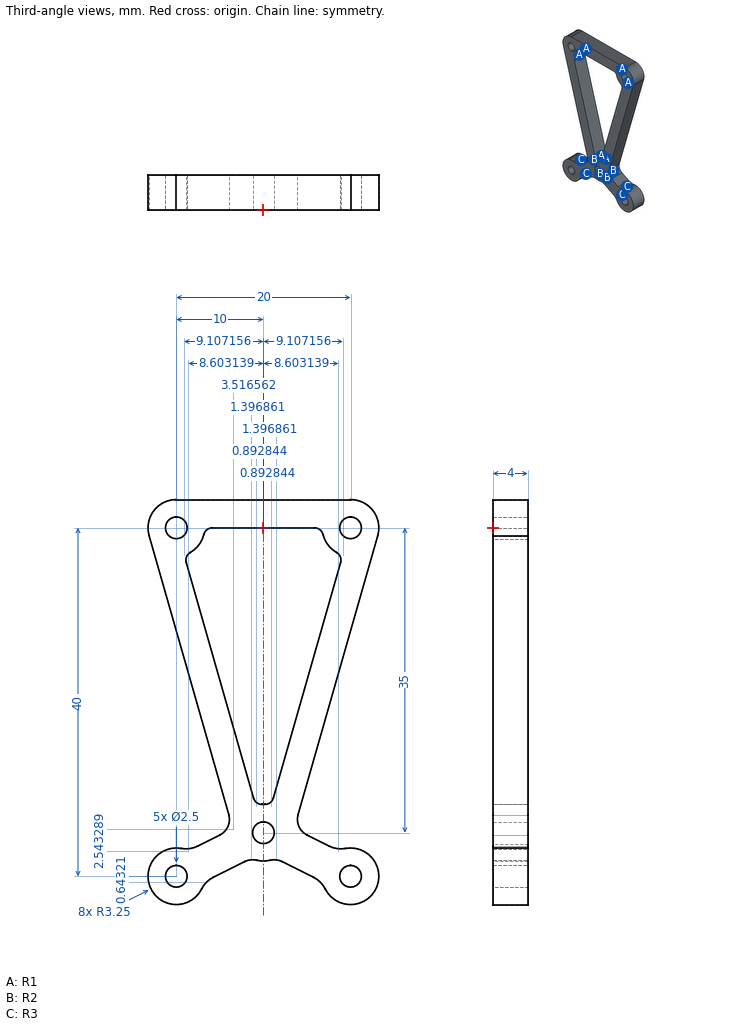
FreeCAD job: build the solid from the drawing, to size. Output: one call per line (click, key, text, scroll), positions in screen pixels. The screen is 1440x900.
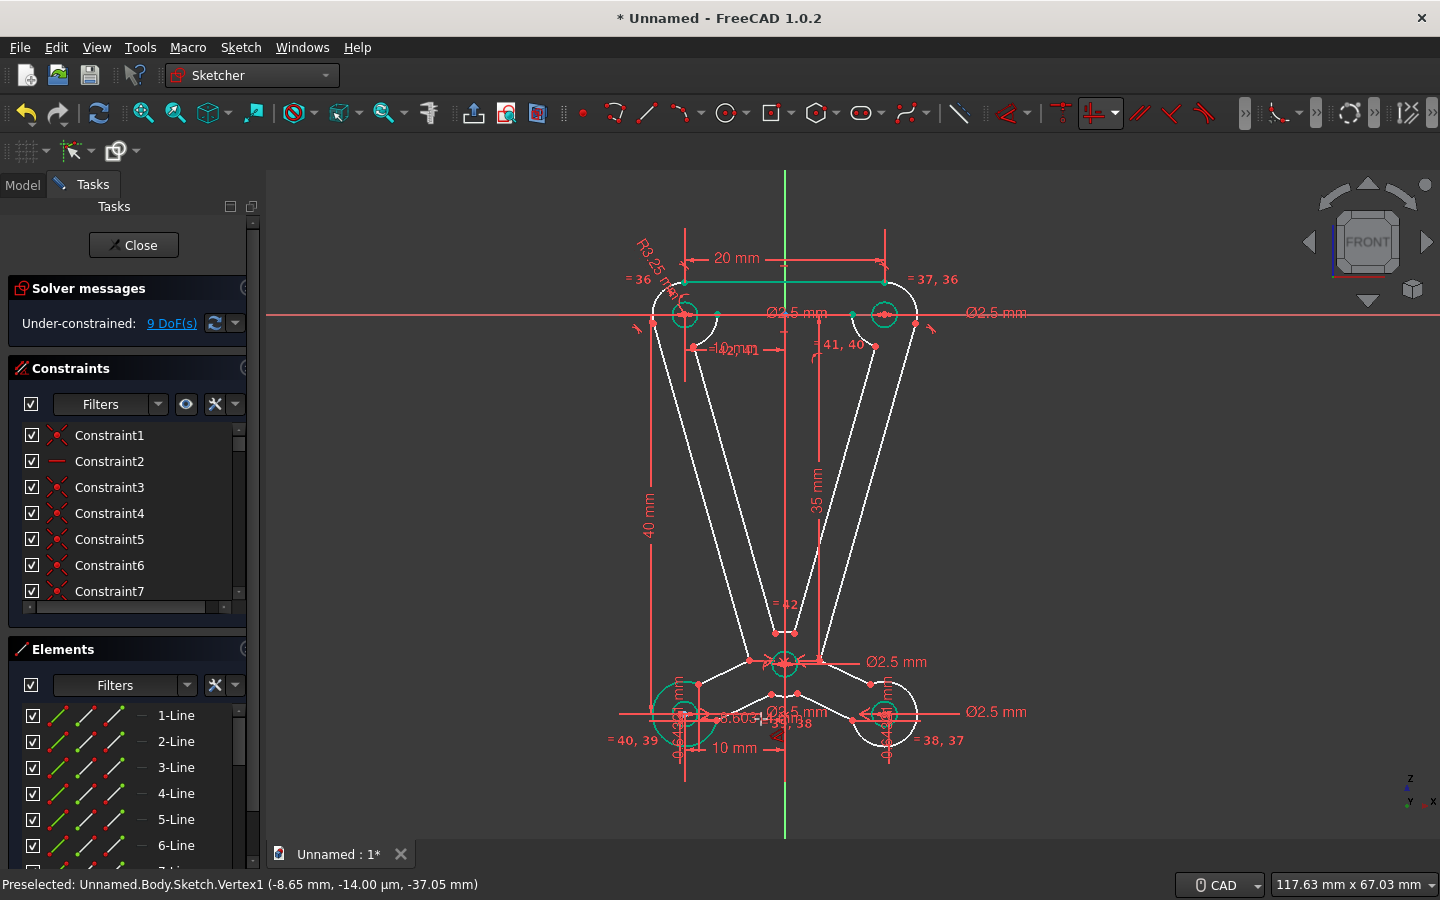
click(750, 661)
click(767, 233)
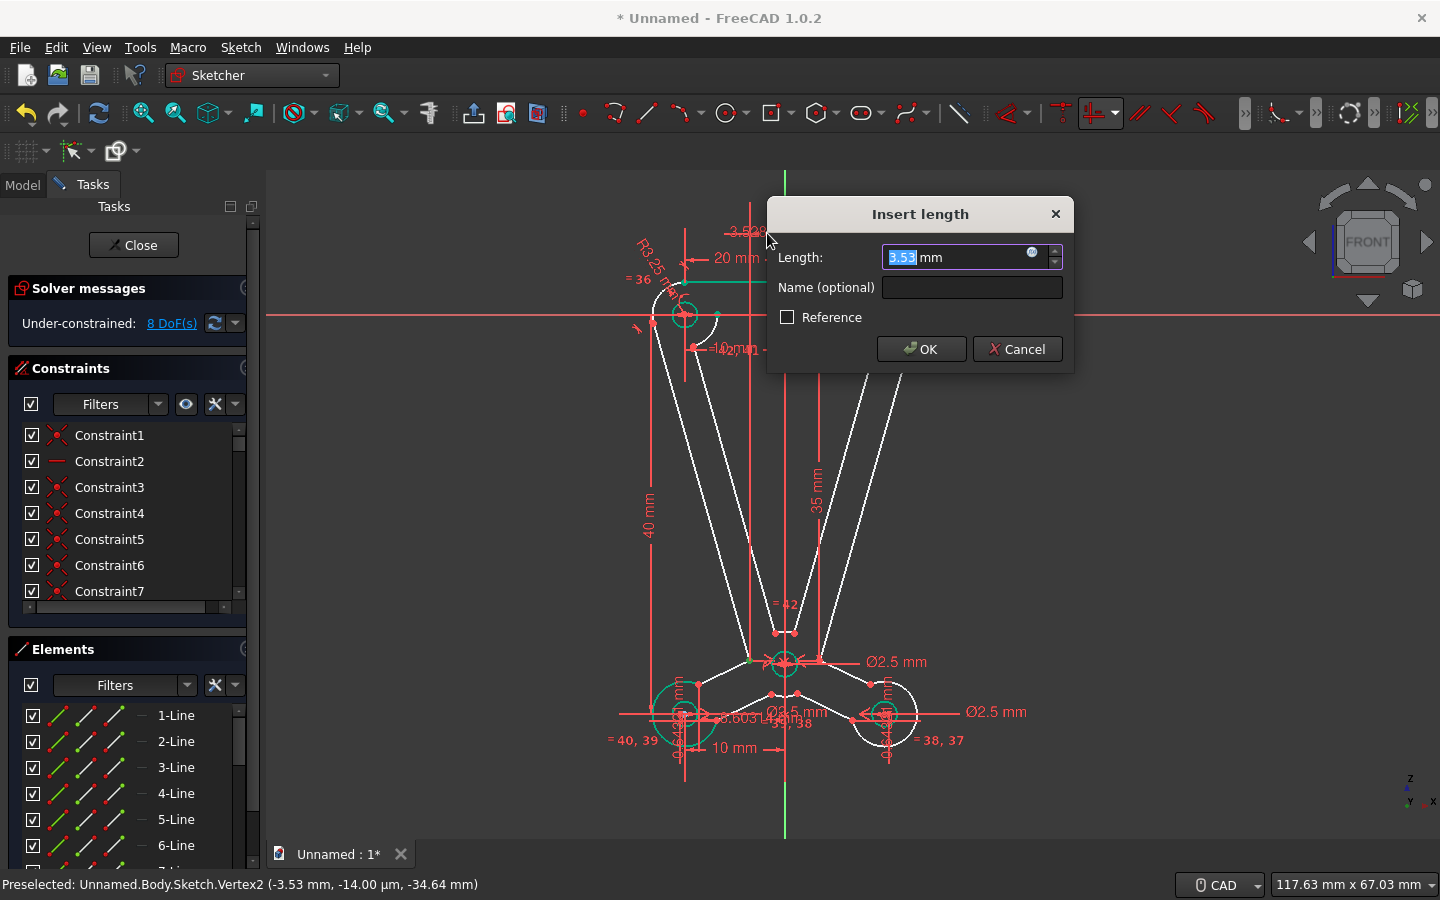
text(3.516562)
key(Return)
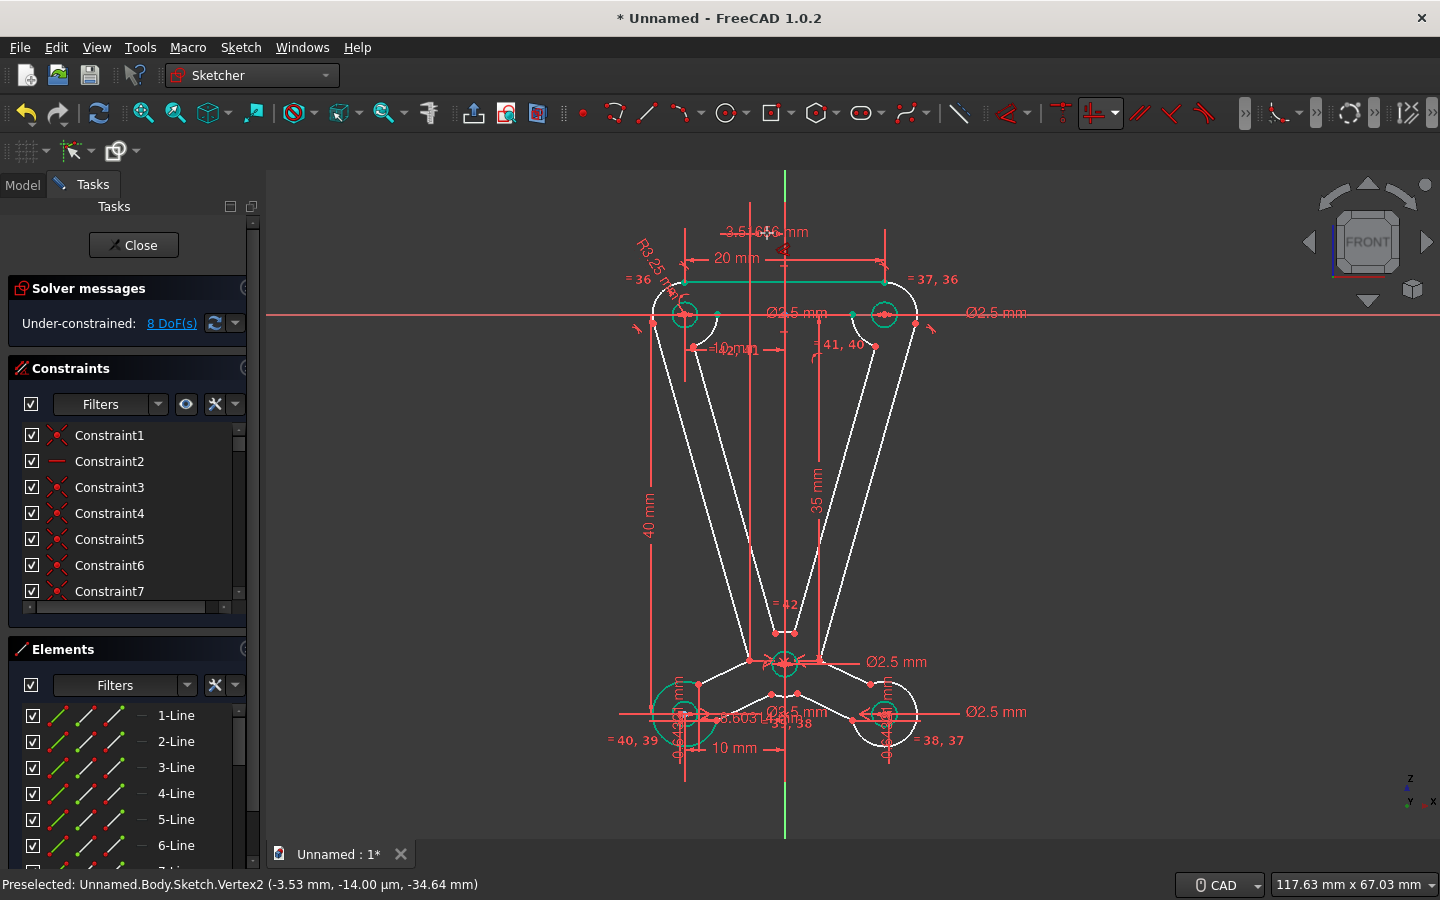
click(871, 685)
click(828, 257)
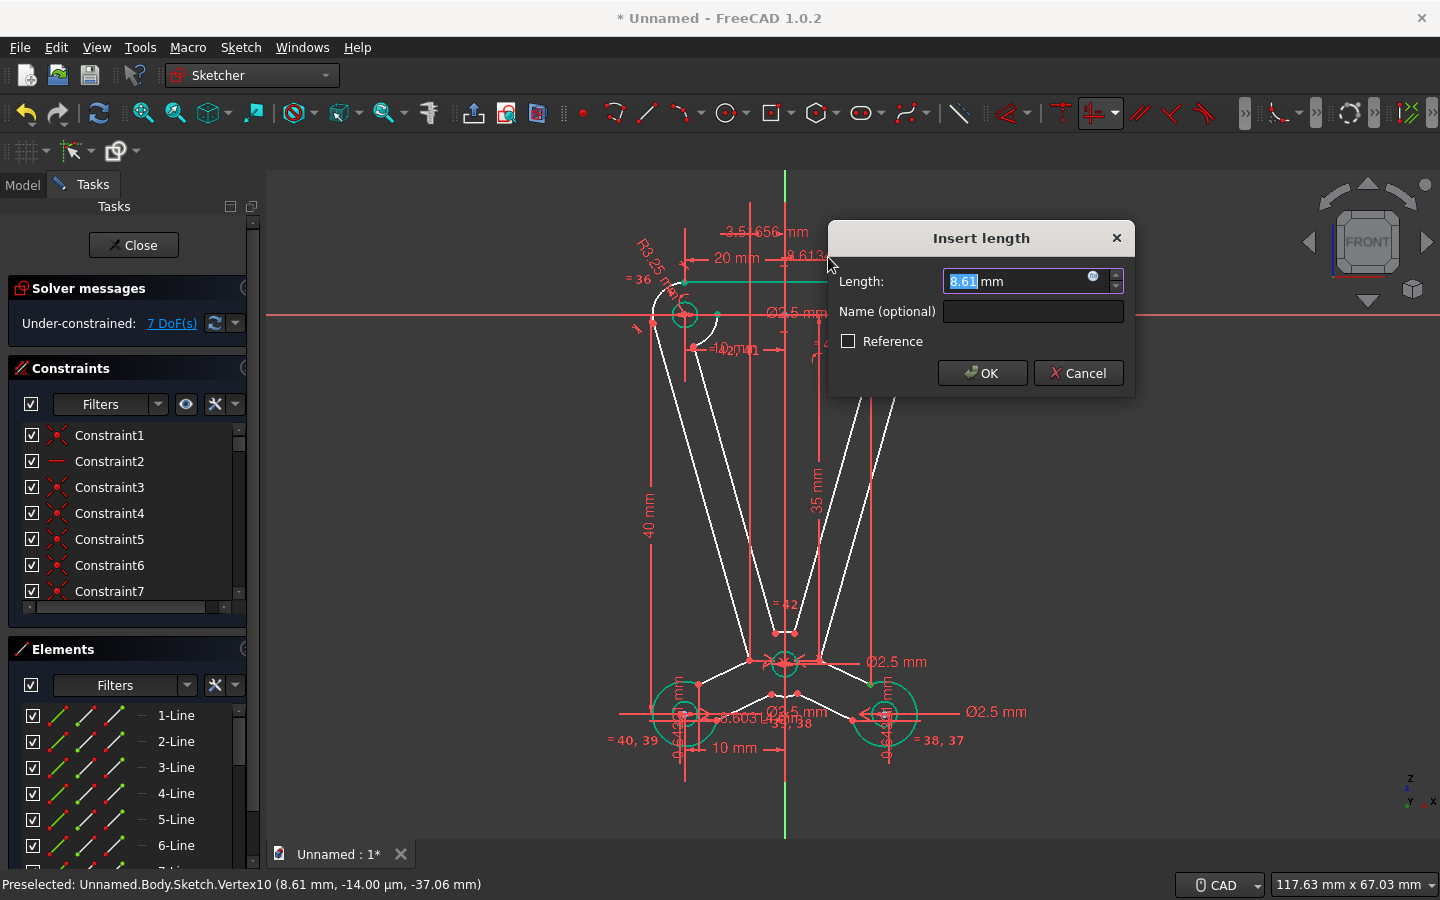
text(8.603139)
key(Return)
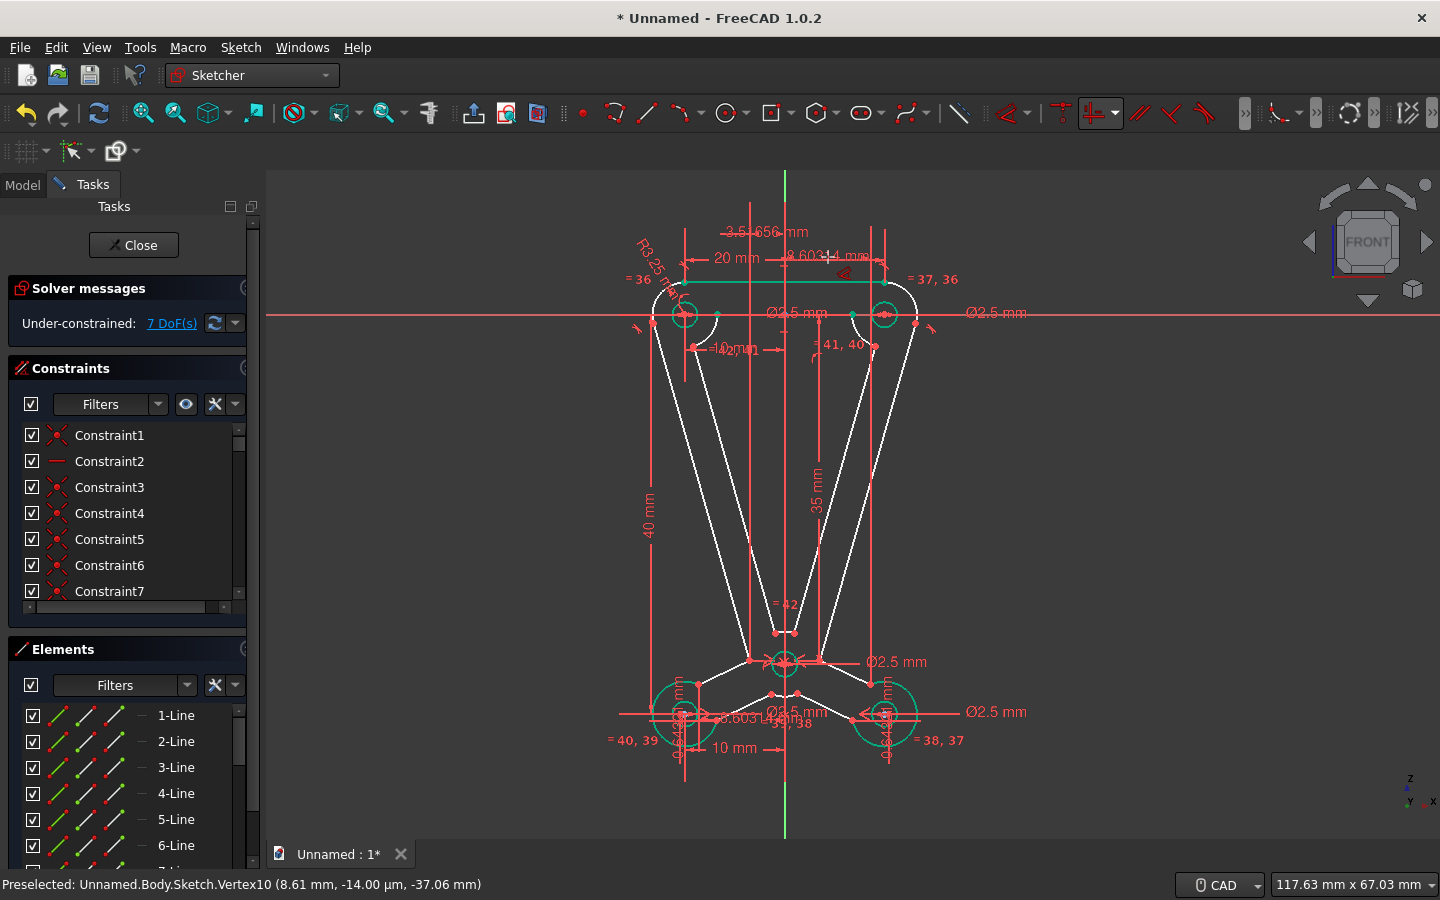
scroll(798, 694, up, 6)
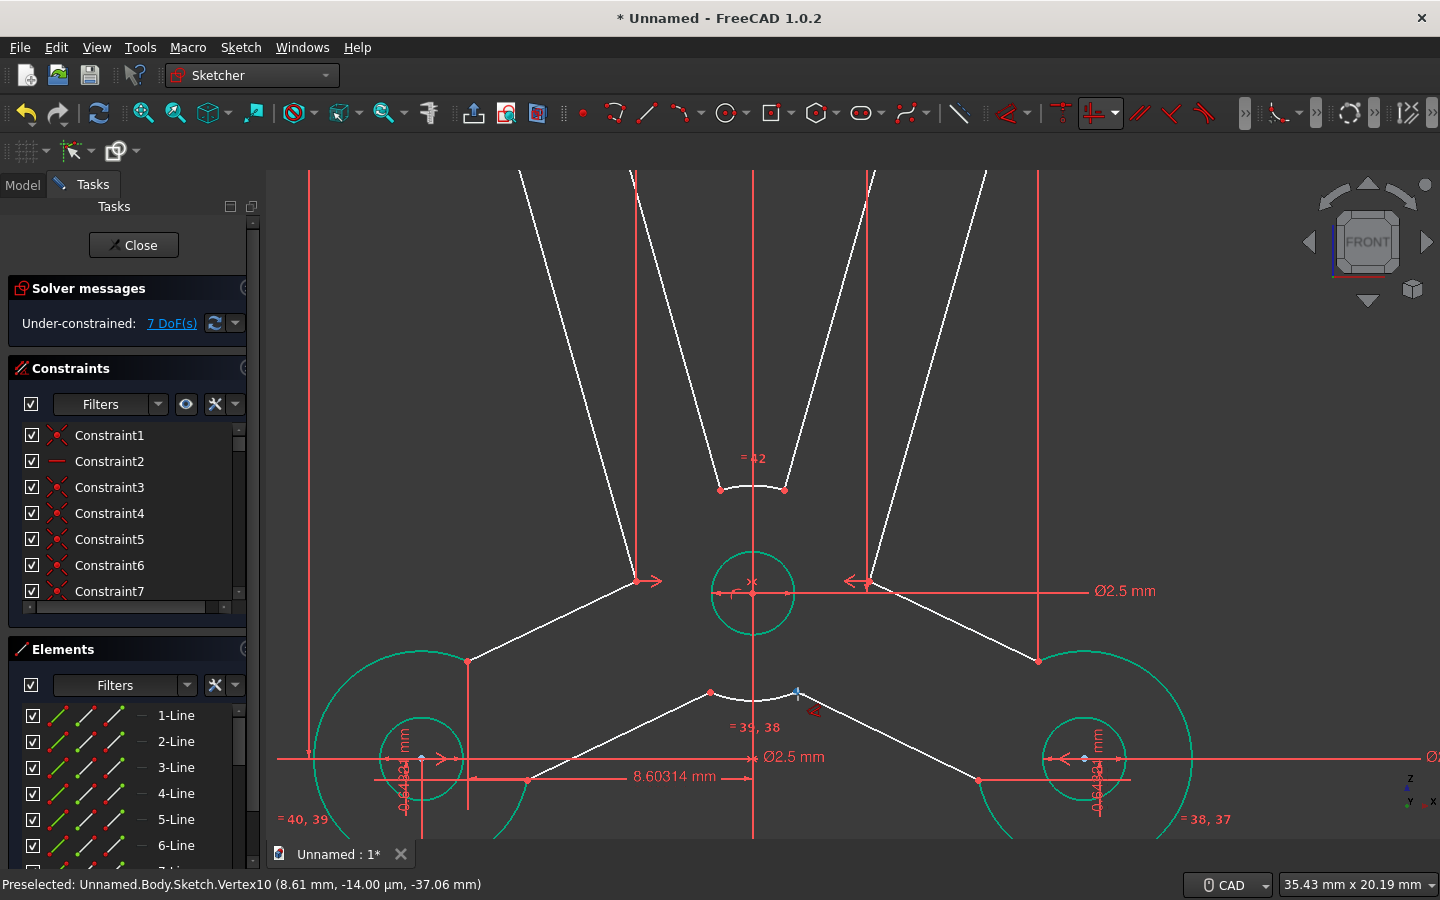
click(797, 692)
click(775, 726)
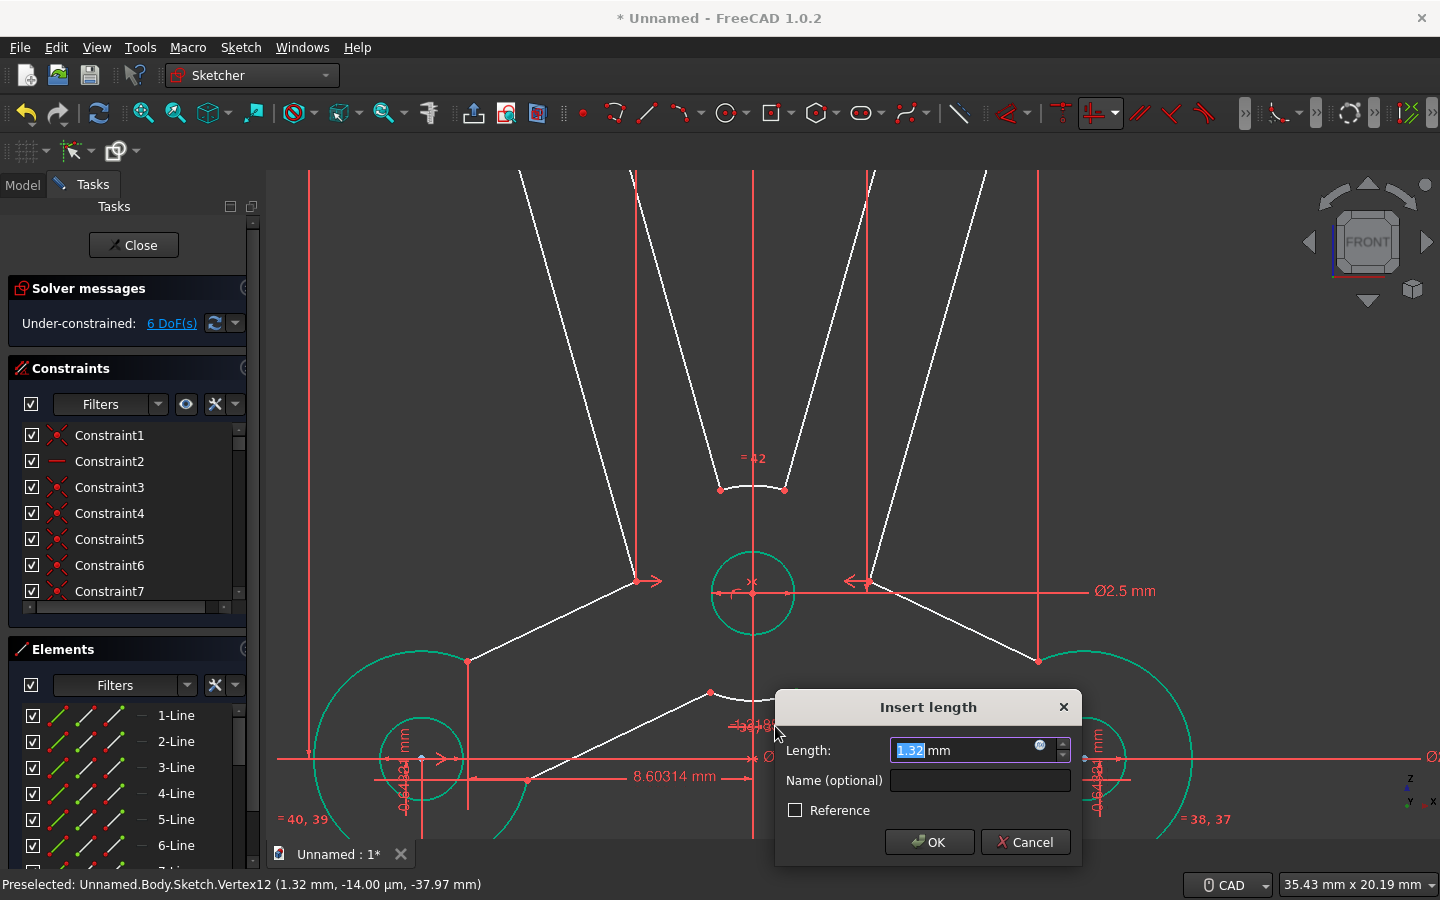
text(1.396861)
key(Return)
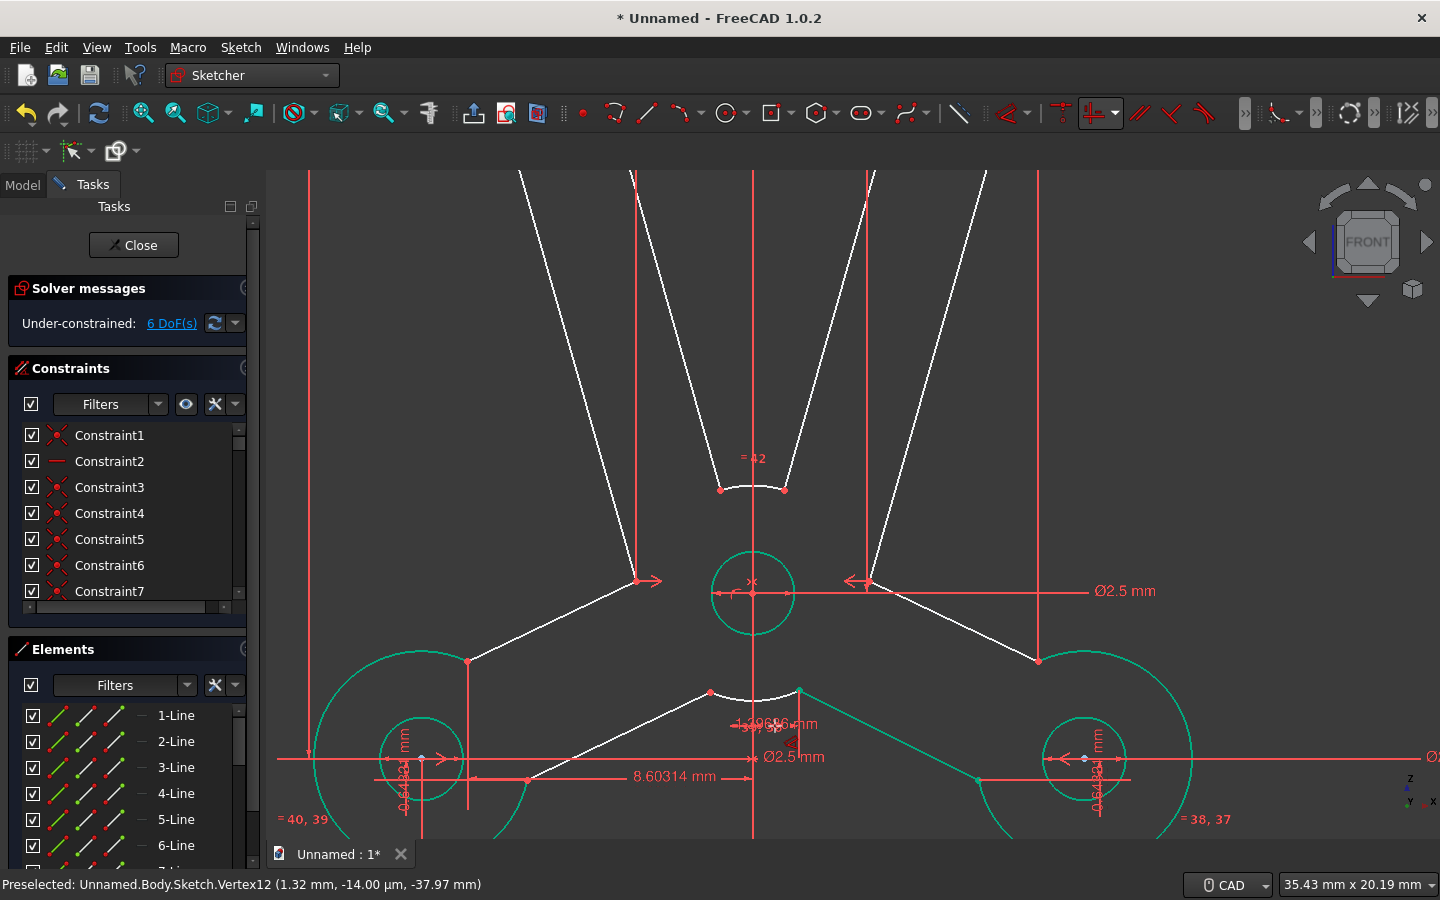
click(711, 692)
click(732, 750)